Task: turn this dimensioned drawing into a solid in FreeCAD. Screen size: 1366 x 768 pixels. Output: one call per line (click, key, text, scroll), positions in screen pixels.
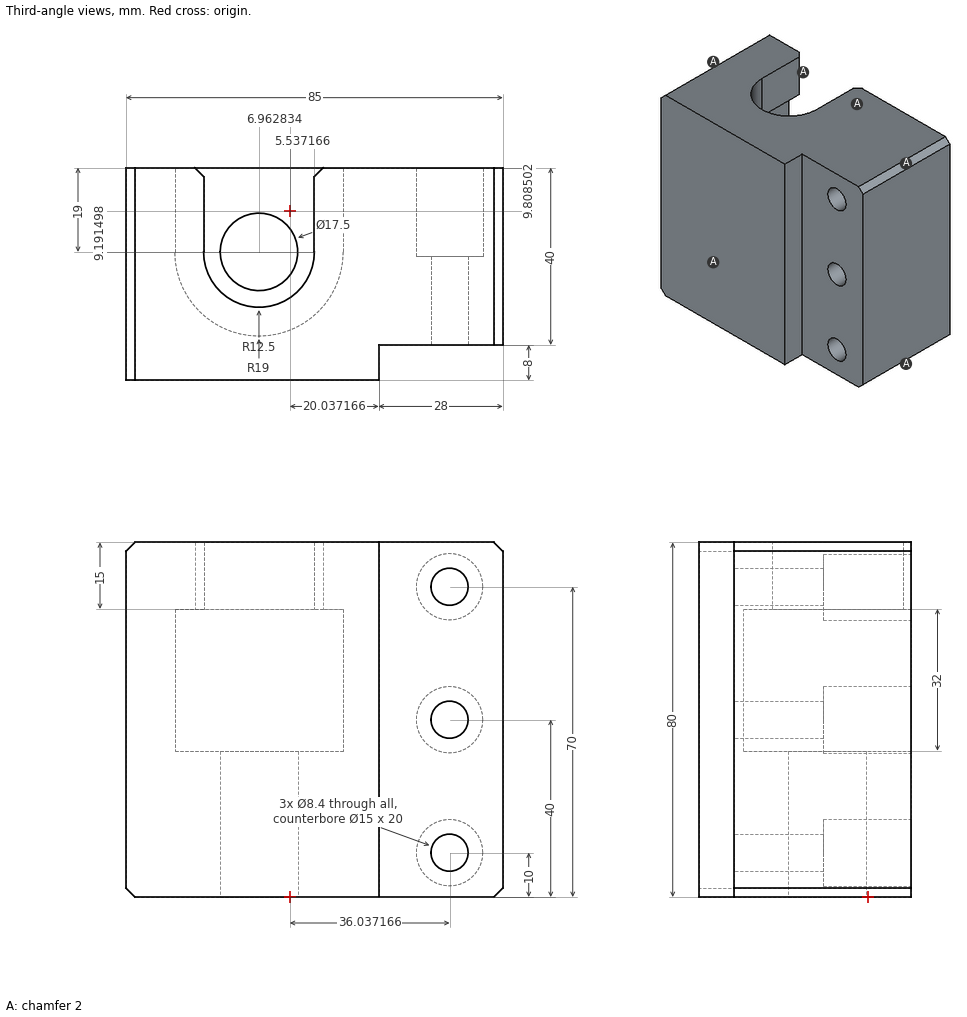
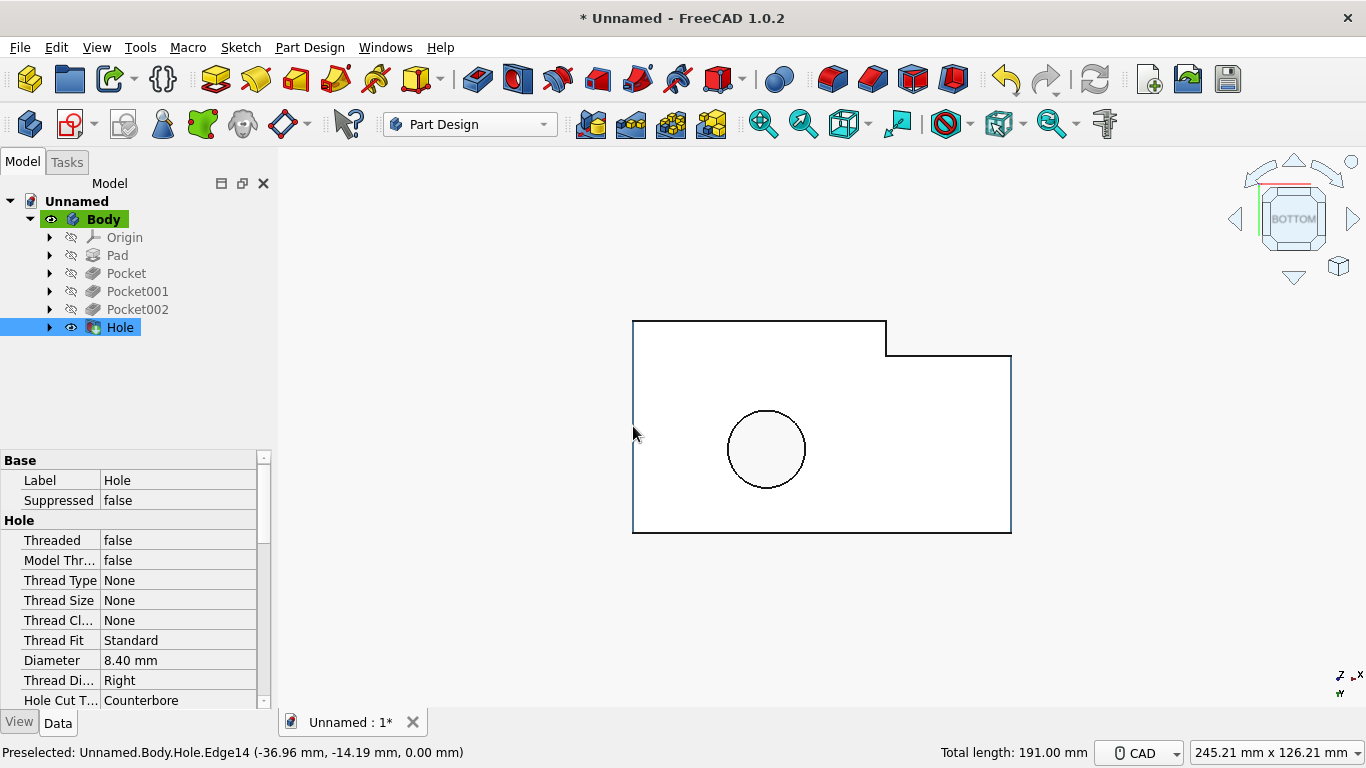
key(4)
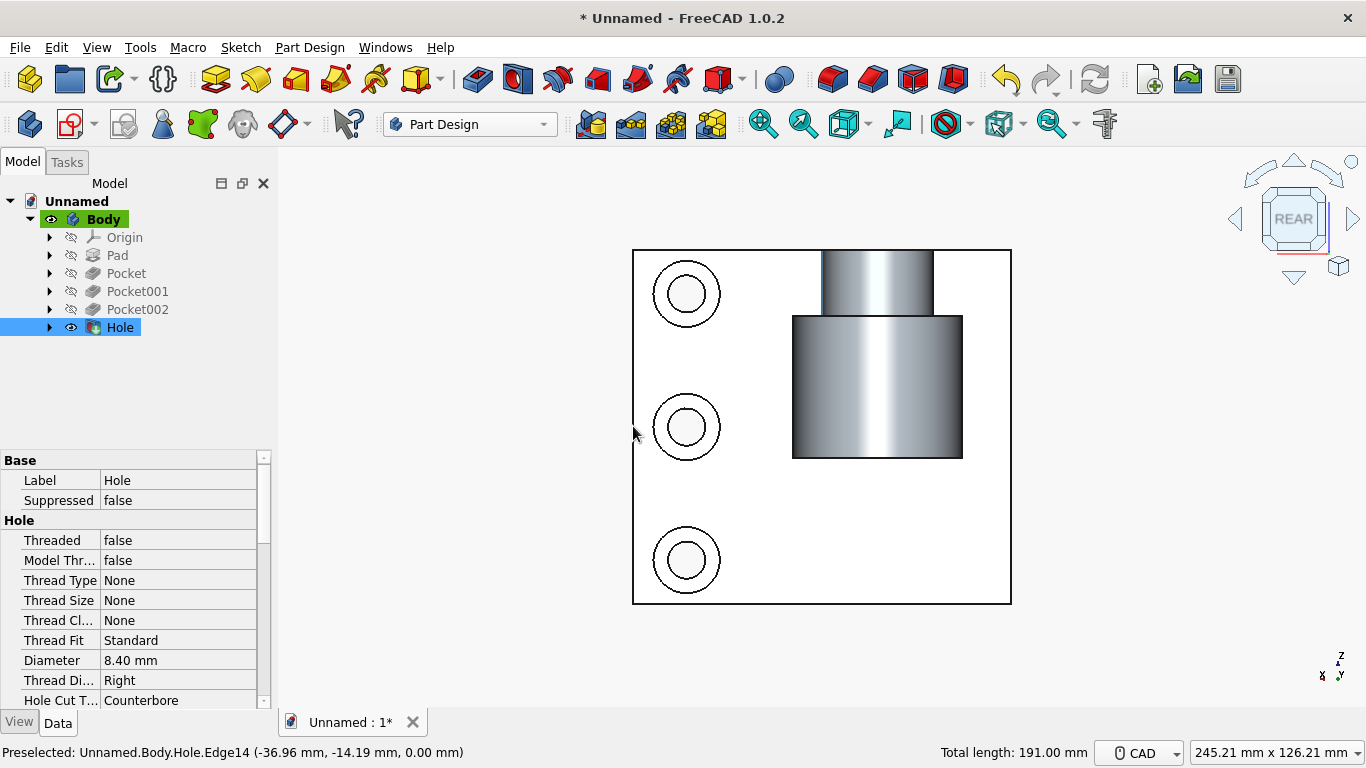
click(933, 282, ctrl)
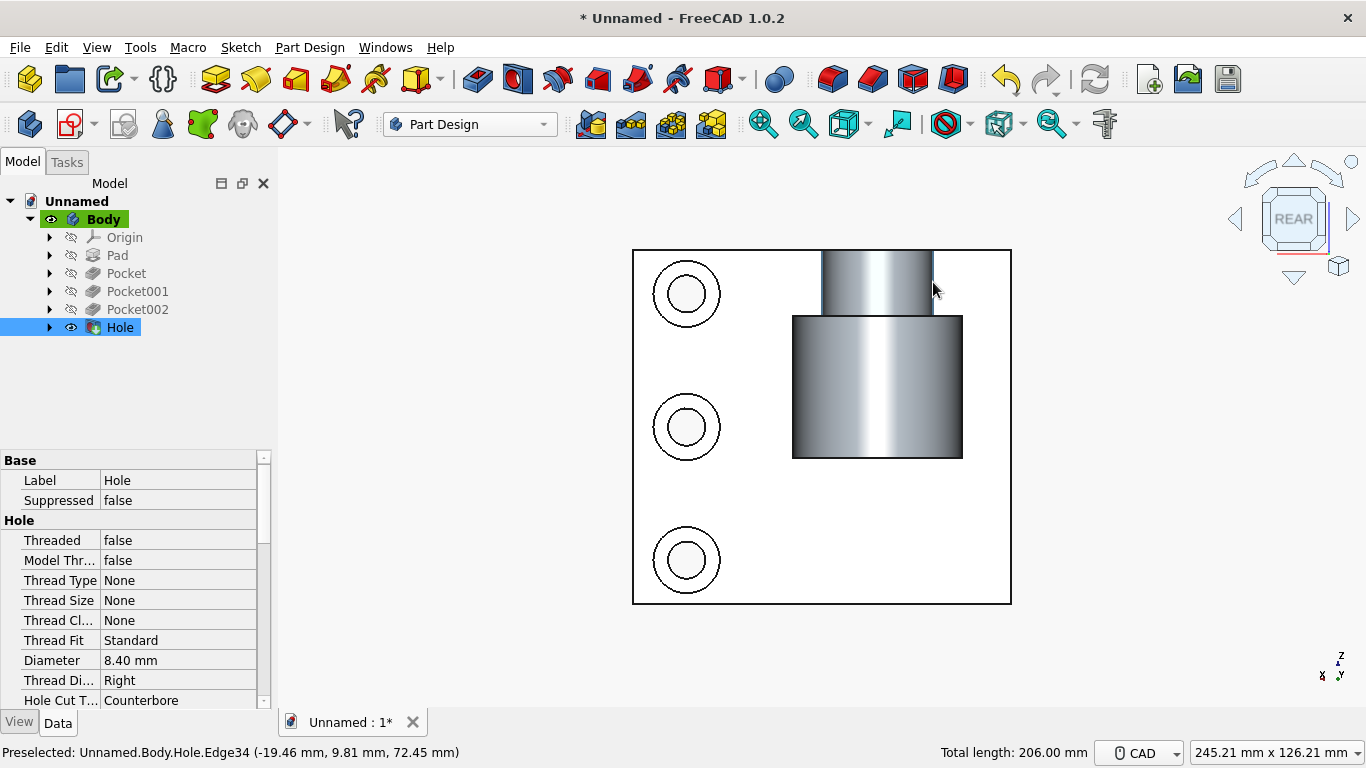
click(874, 80)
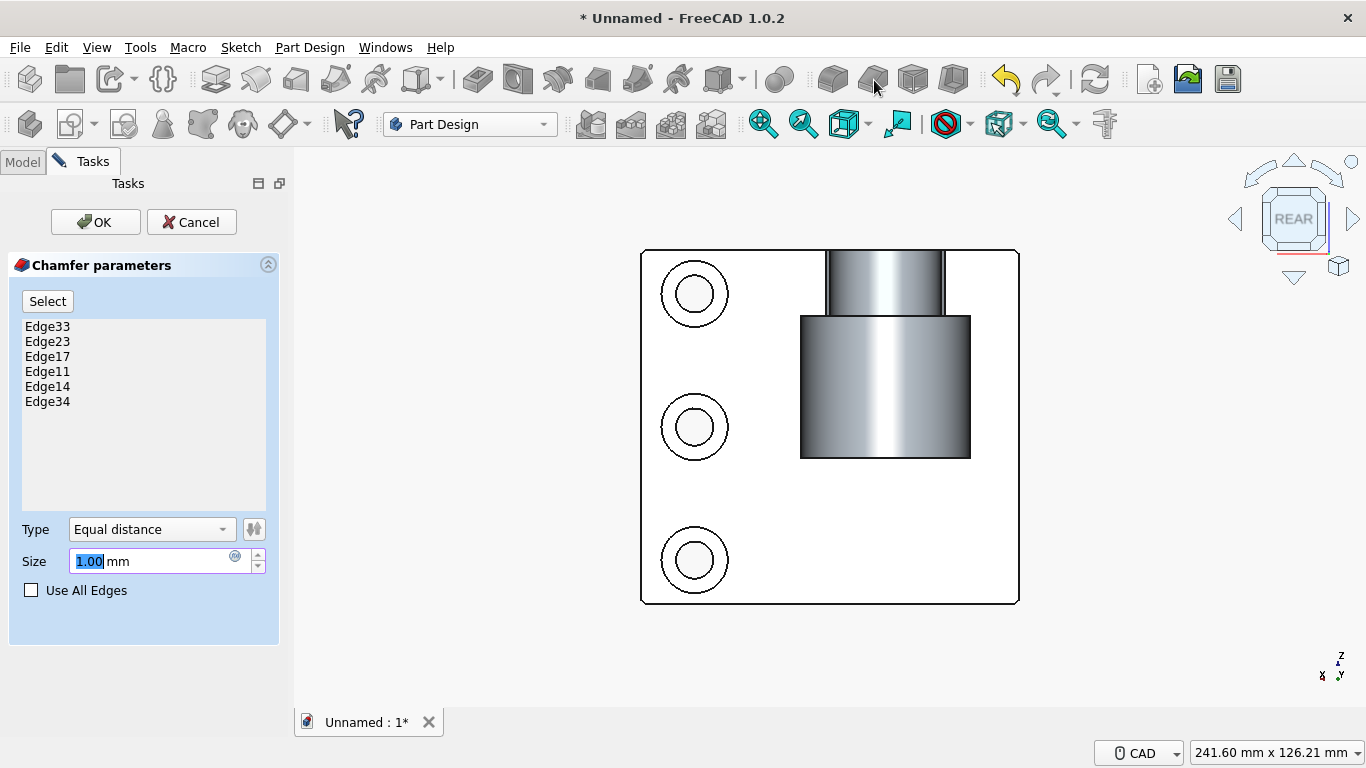
text(2)
key(Tab)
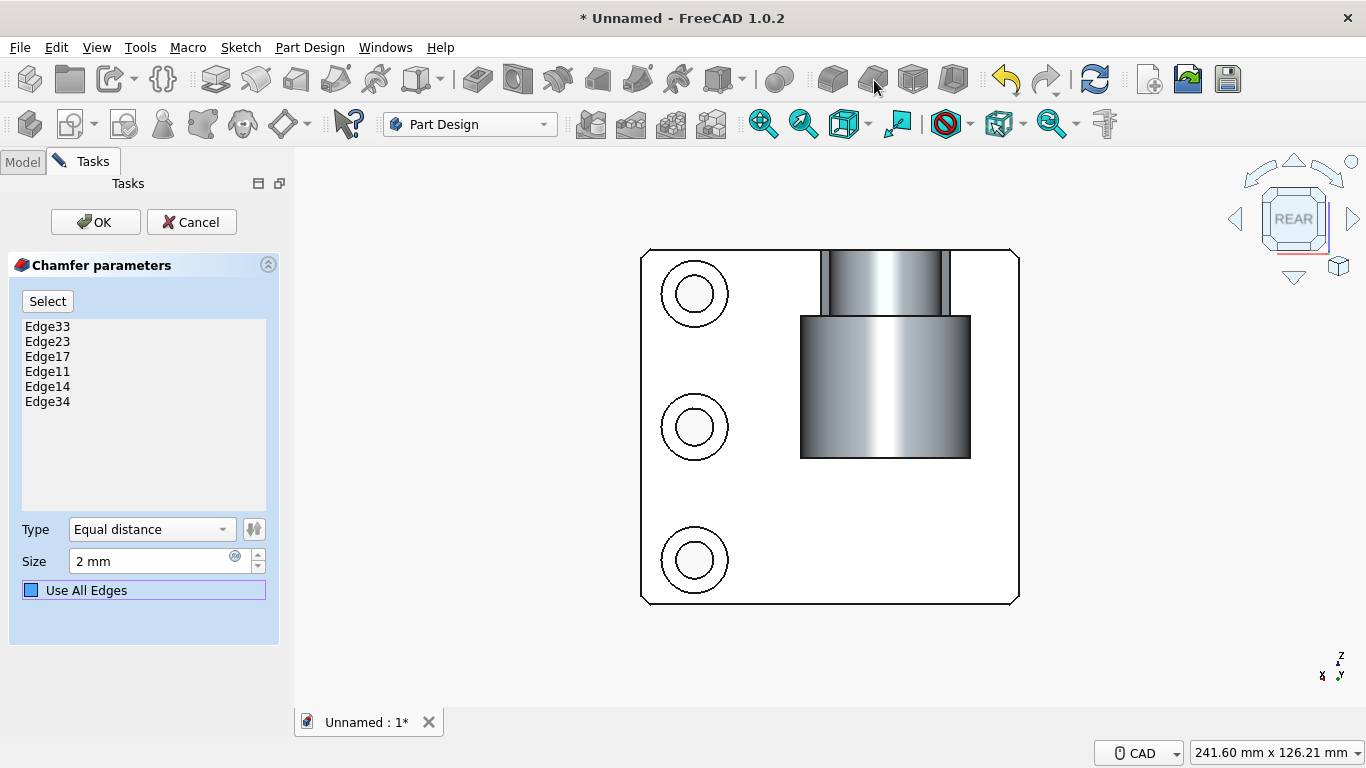
click(96, 222)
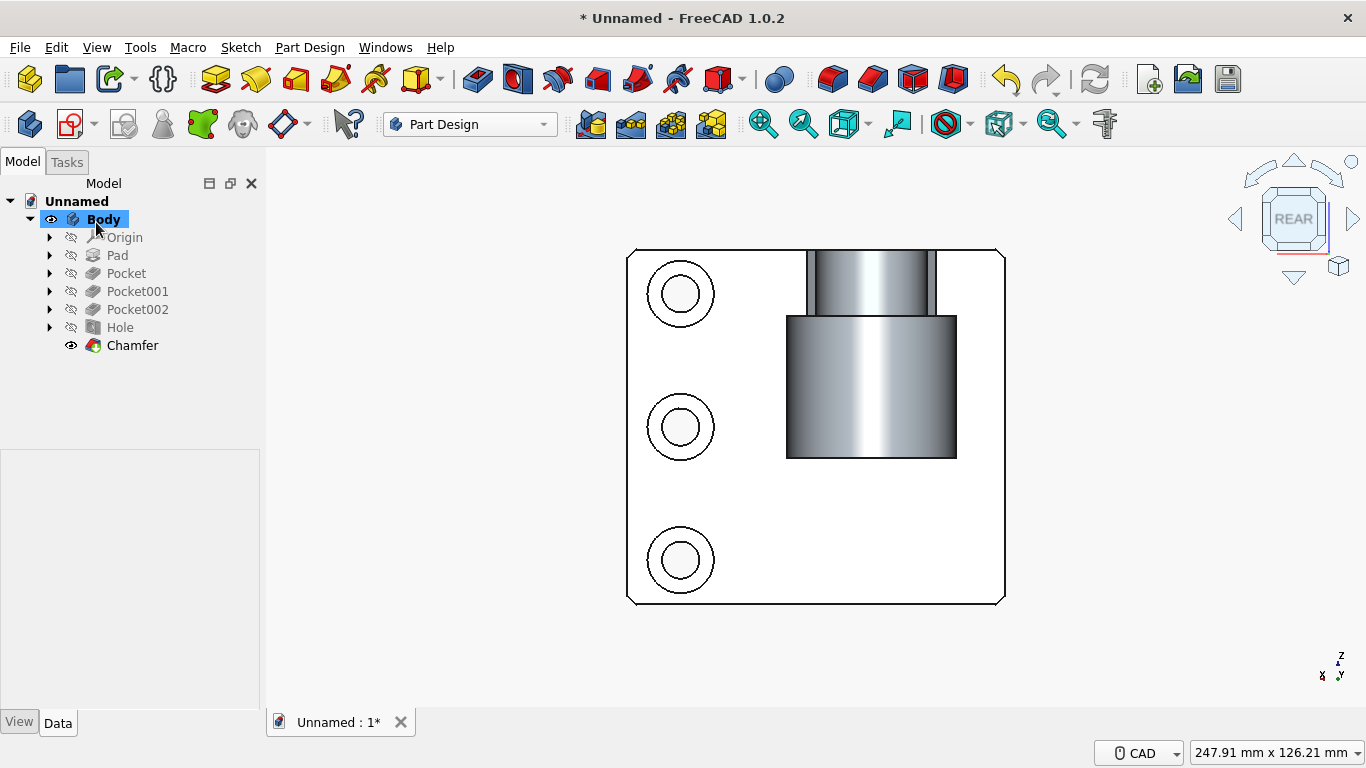
key(0)